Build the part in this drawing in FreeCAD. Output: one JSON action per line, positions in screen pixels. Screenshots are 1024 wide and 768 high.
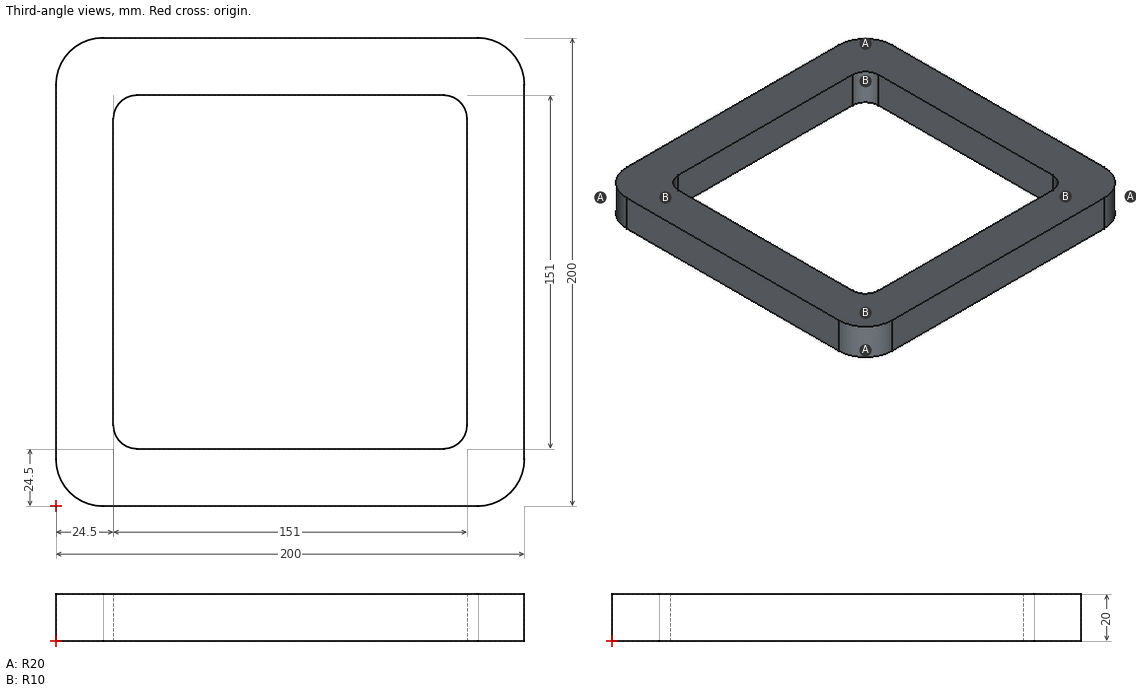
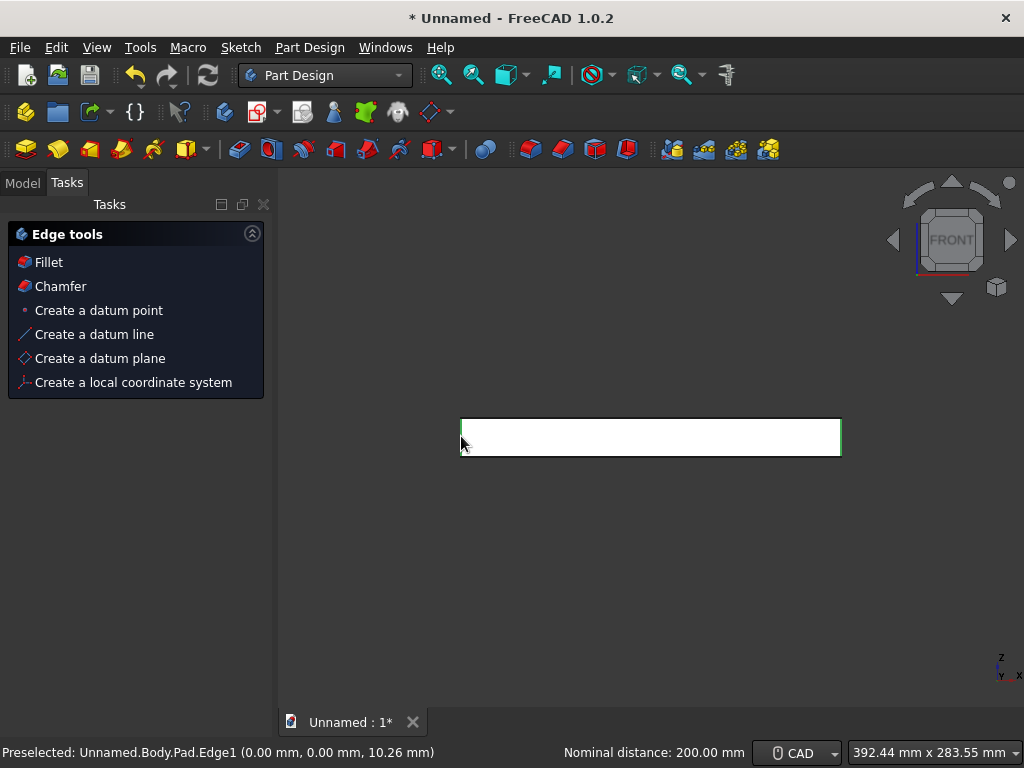
{"action": "key", "text": "3"}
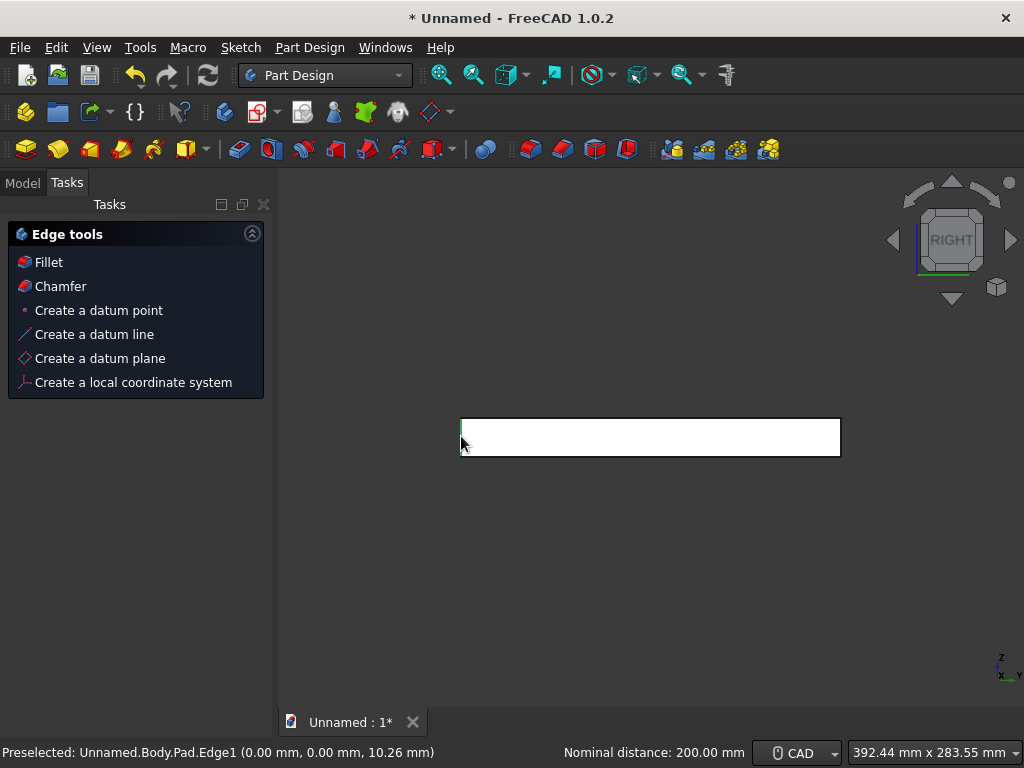
{"action": "left_click", "coordinate": [841, 436], "text": "ctrl"}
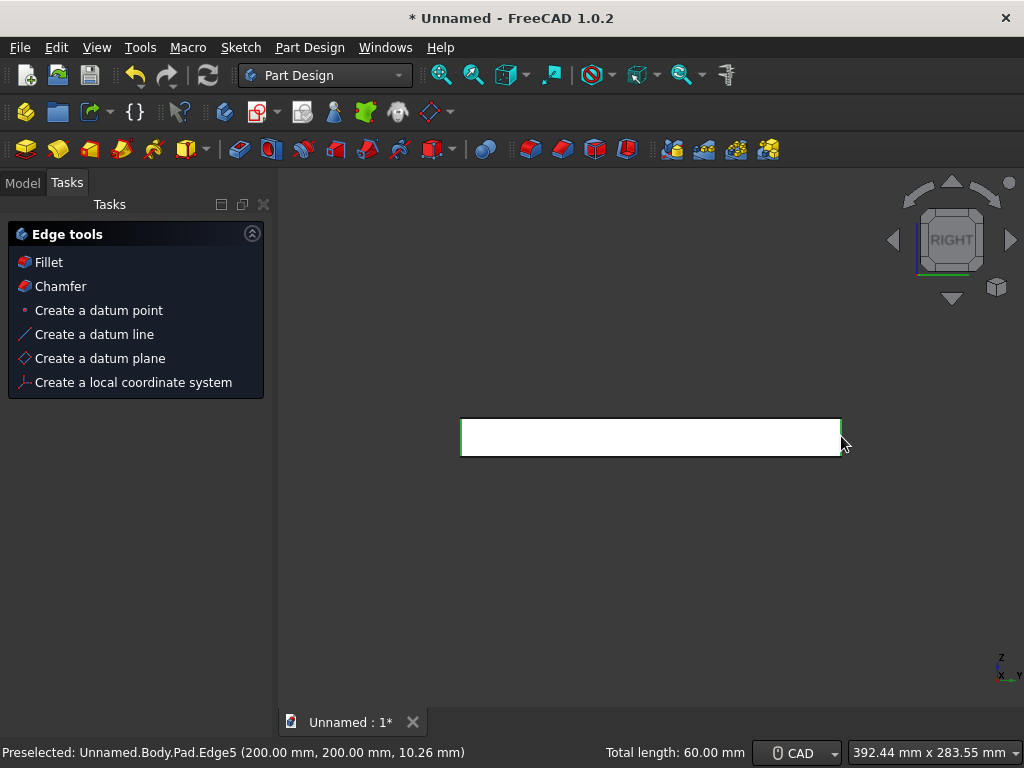
{"action": "key", "text": "5"}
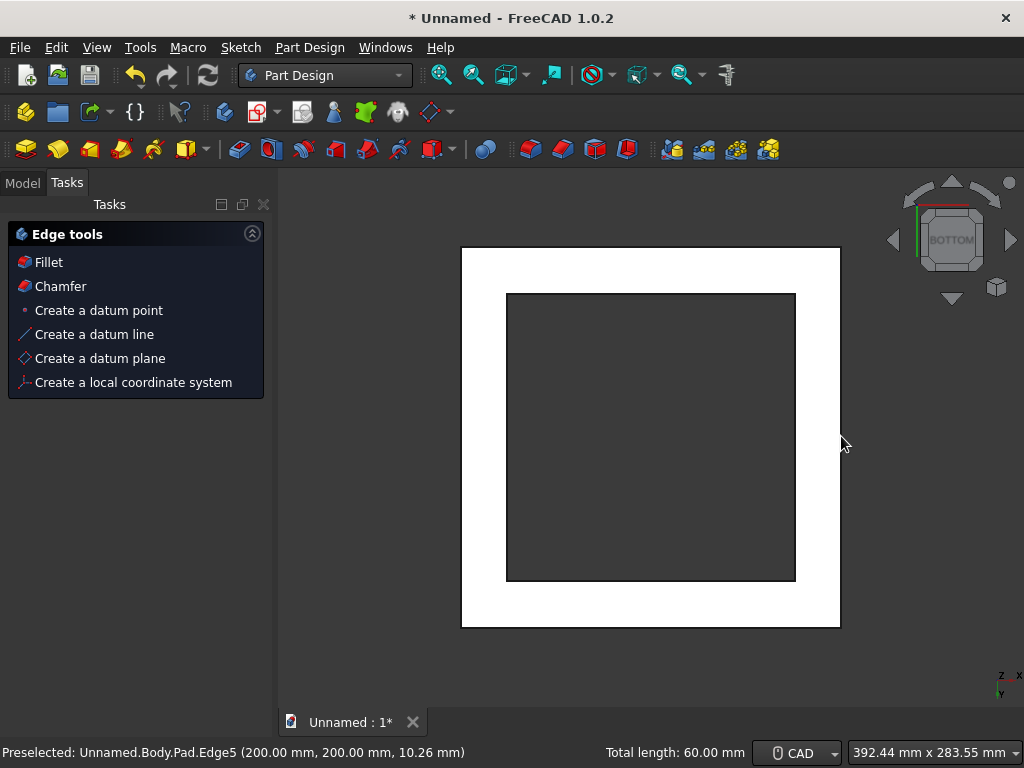
{"action": "key", "text": "4"}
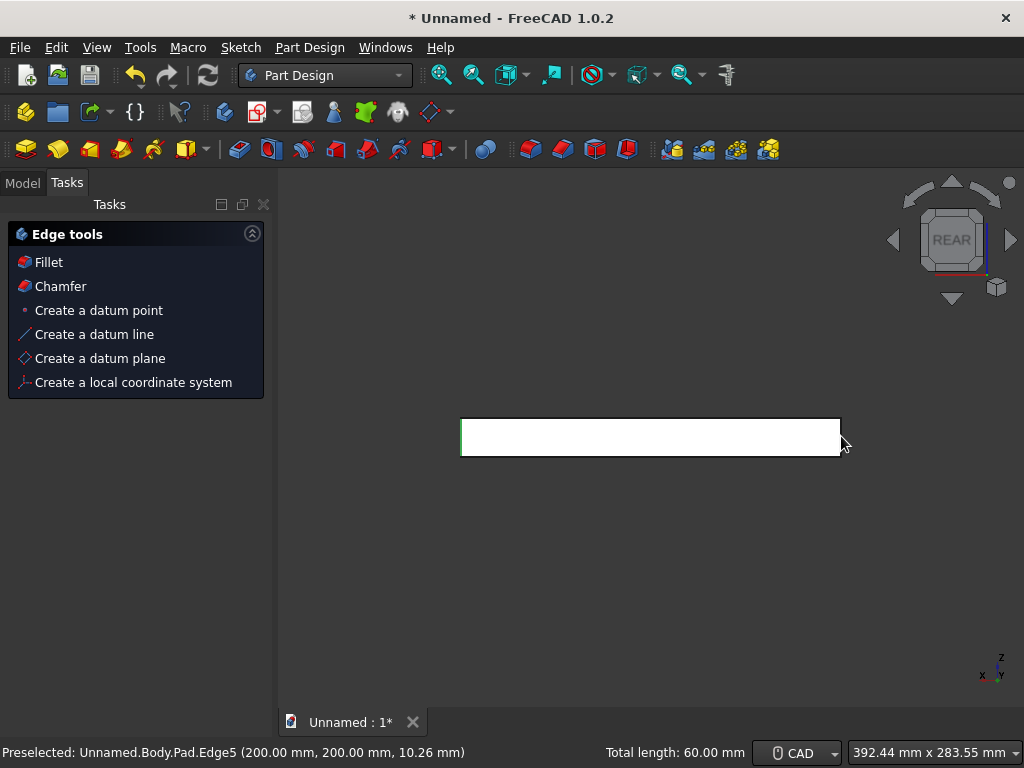
{"action": "left_click", "coordinate": [841, 436], "text": "ctrl"}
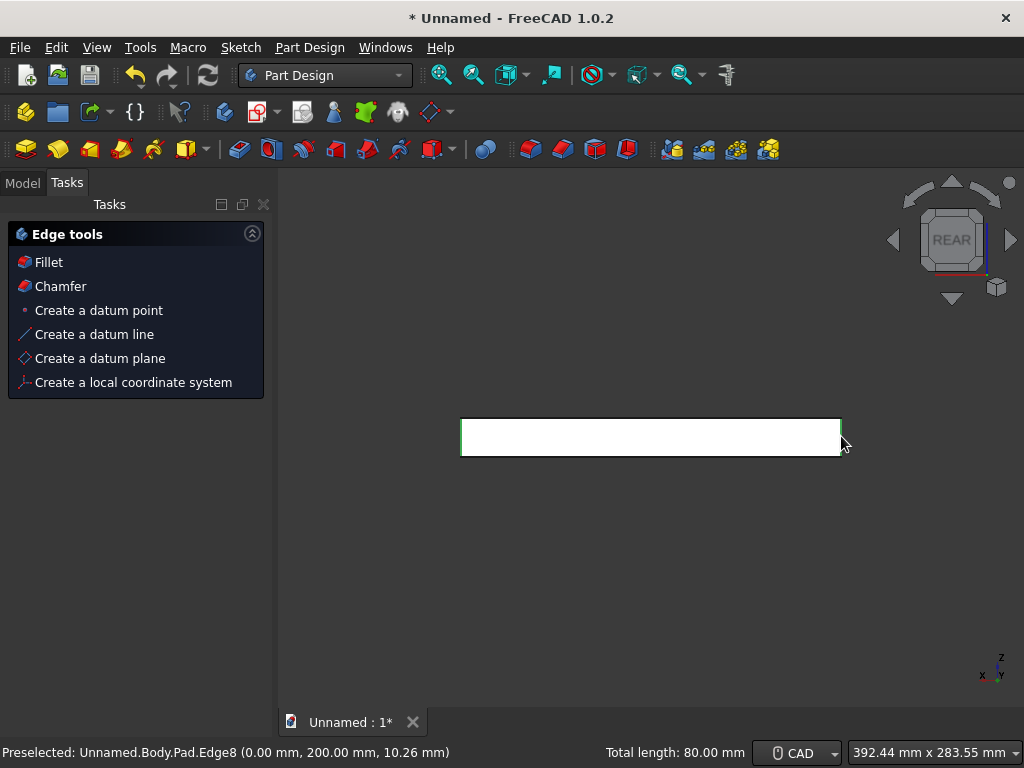
{"action": "left_click", "coordinate": [532, 150]}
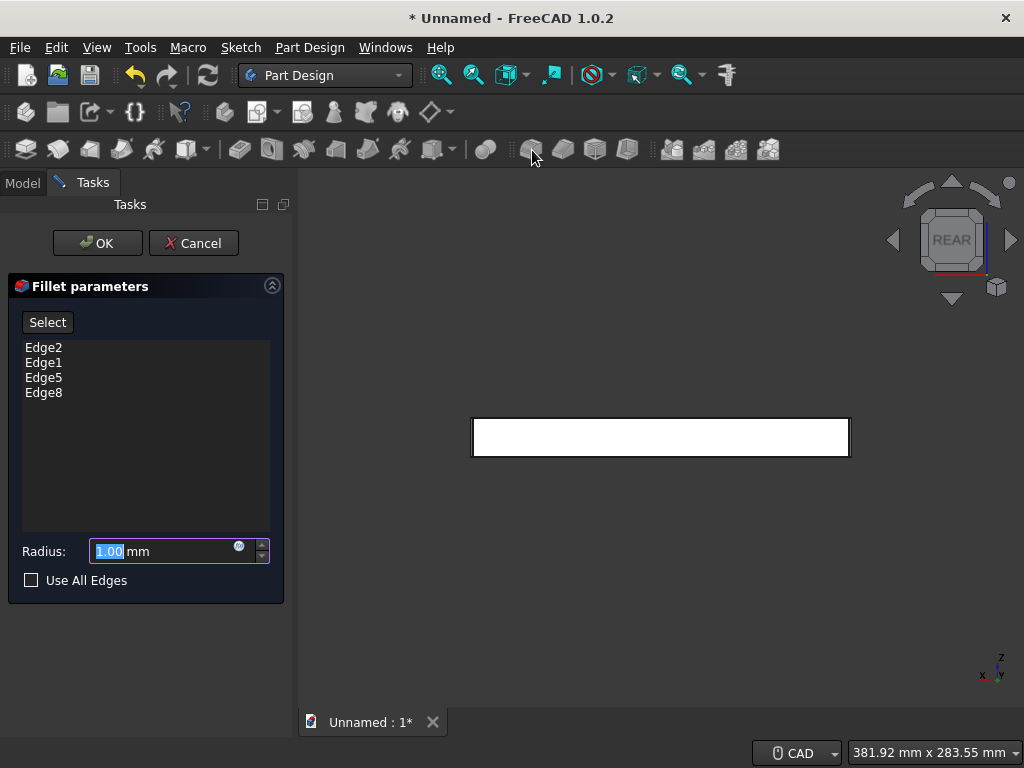
{"action": "type", "text": "20"}
{"action": "key", "text": "Tab"}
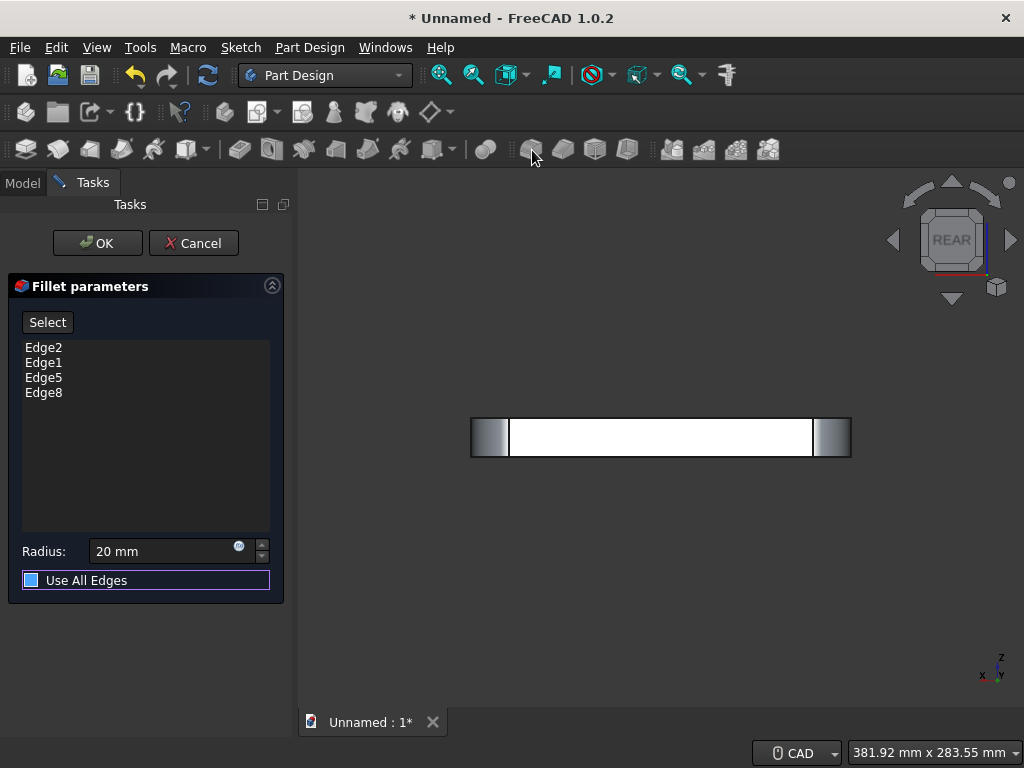
{"action": "left_click", "coordinate": [98, 243]}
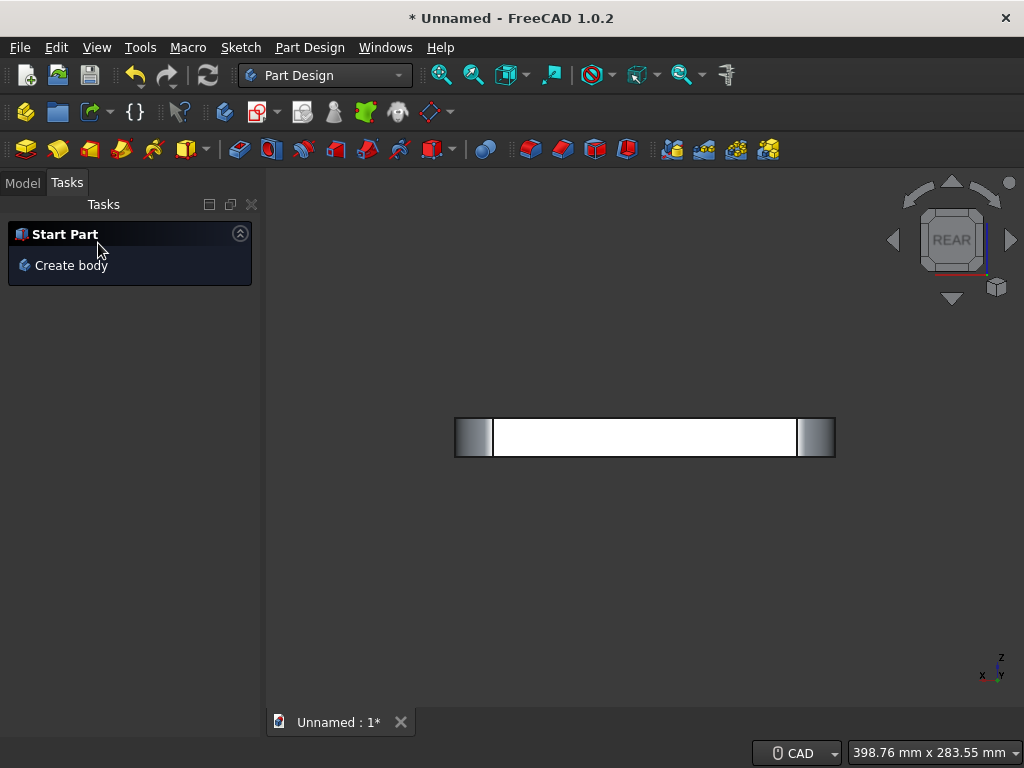
{"action": "key", "text": "0"}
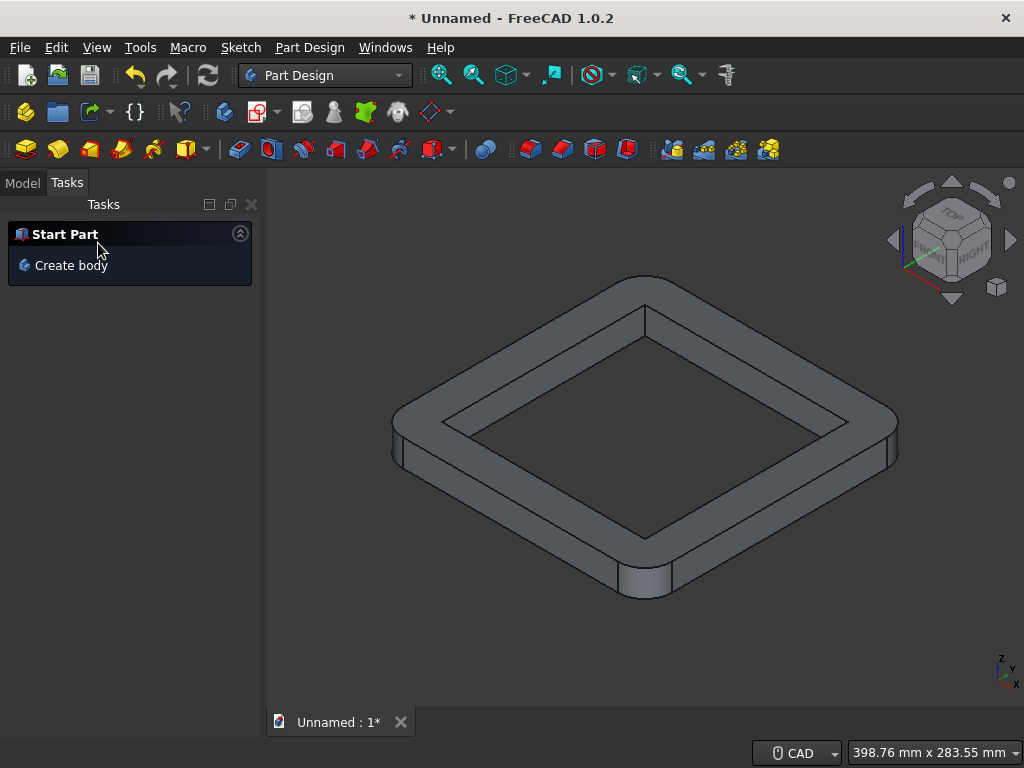
{"action": "key", "text": "2"}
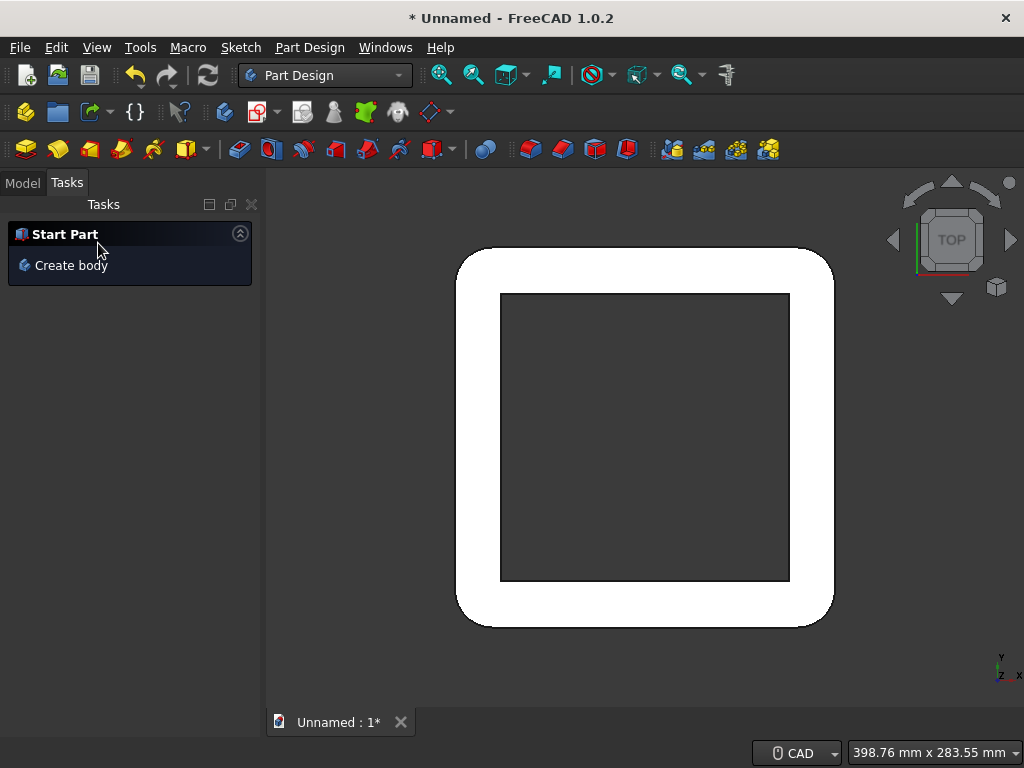
{"action": "key", "text": "1"}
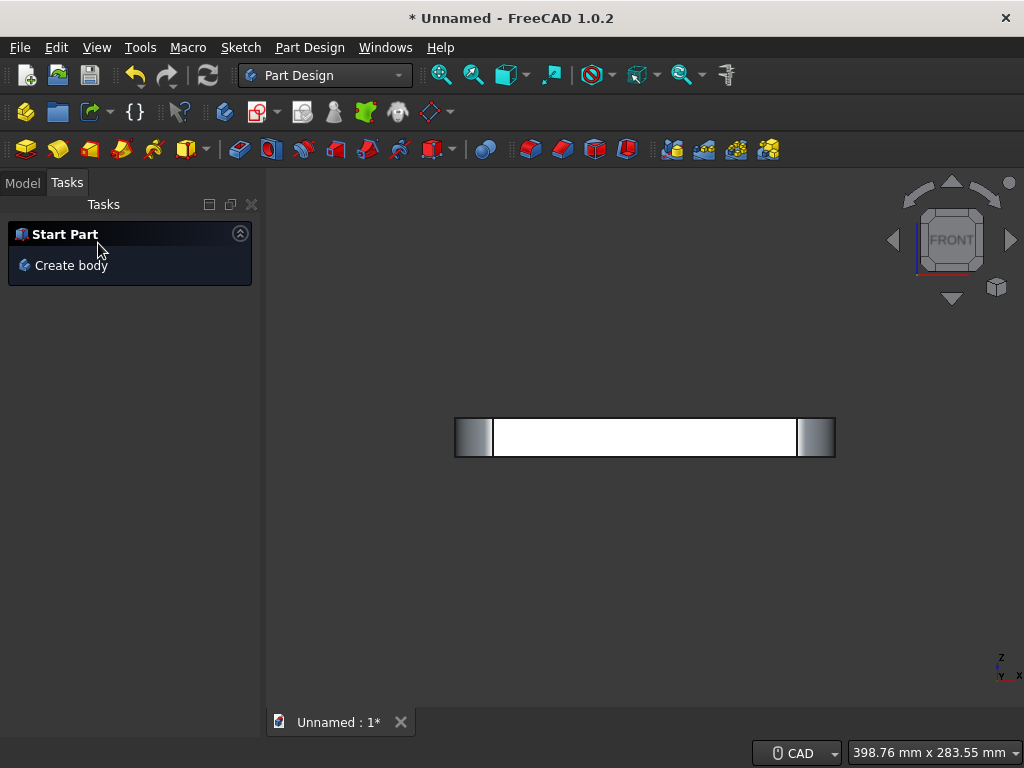
{"action": "key", "text": "3"}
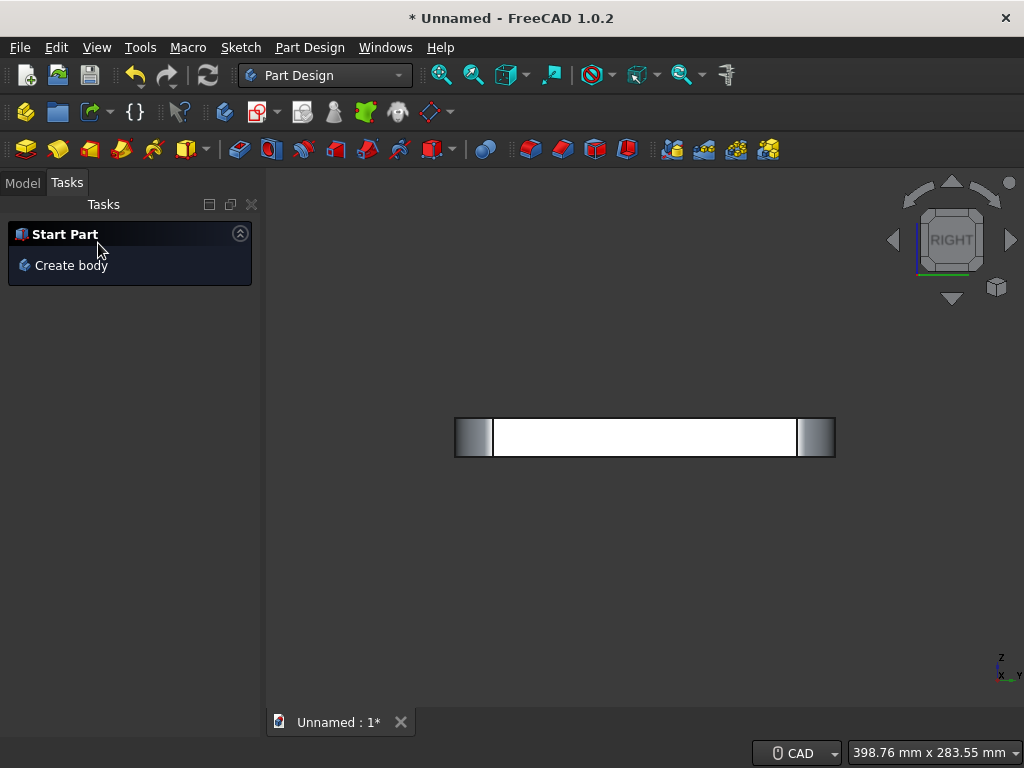
{"action": "key", "text": "5"}